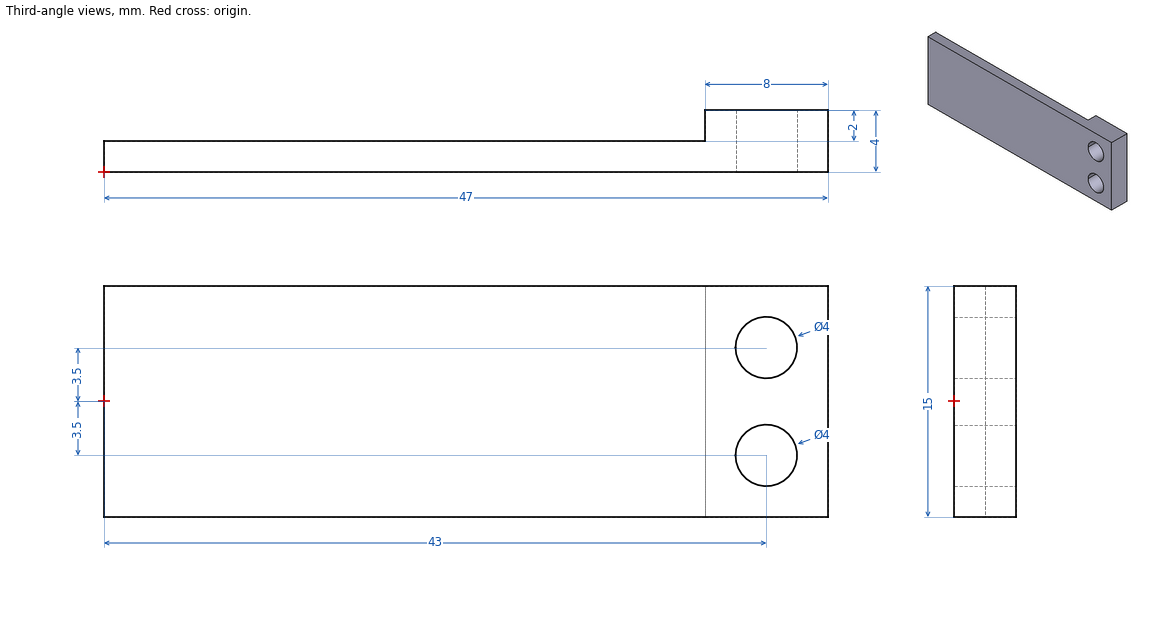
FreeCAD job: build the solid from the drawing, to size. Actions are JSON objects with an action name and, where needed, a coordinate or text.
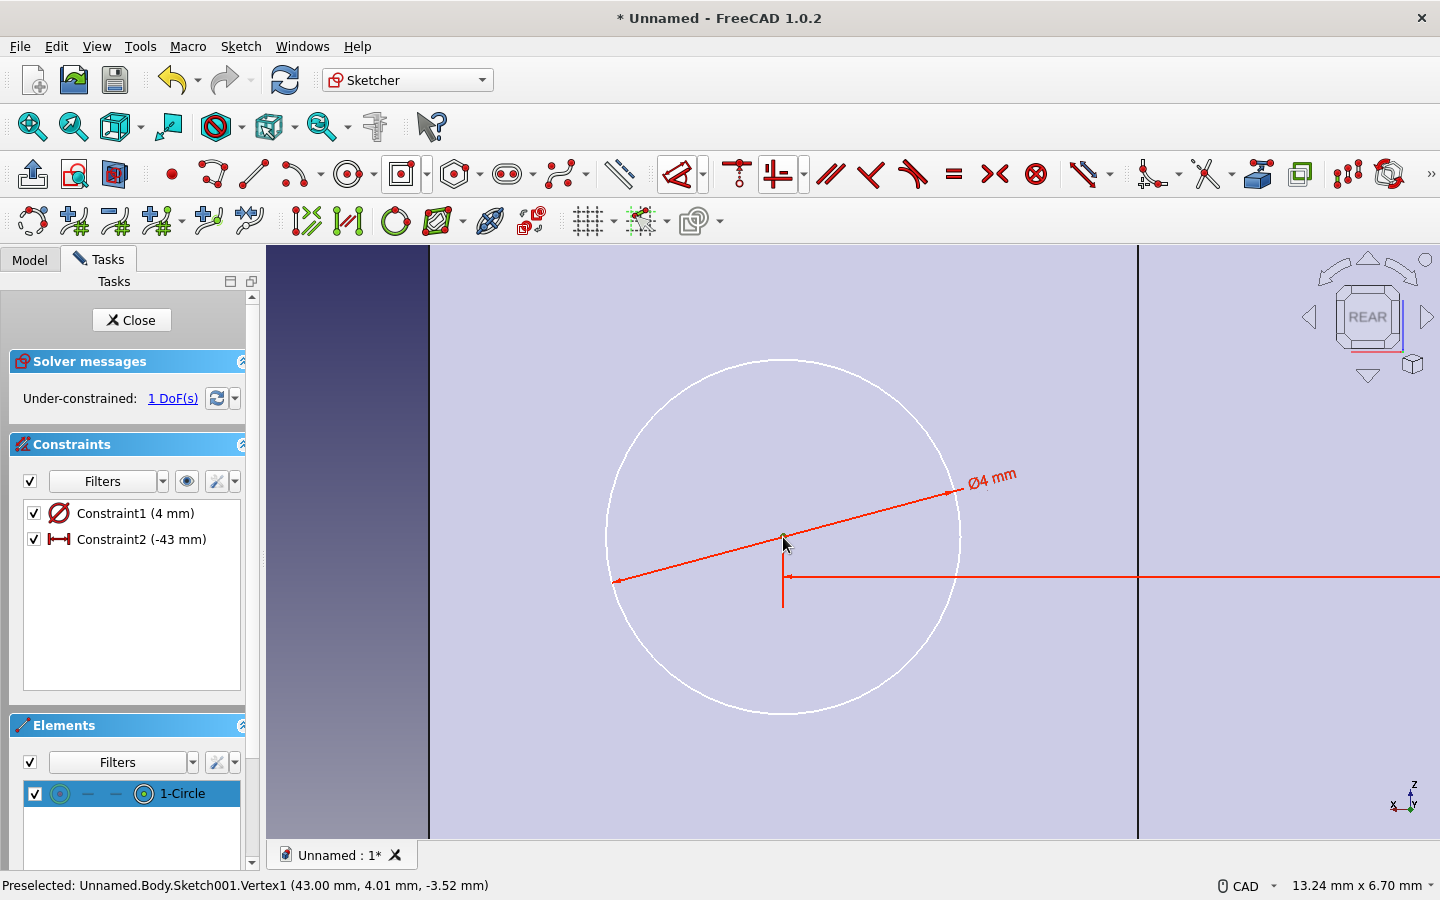
{"action": "left_click", "coordinate": [702, 174]}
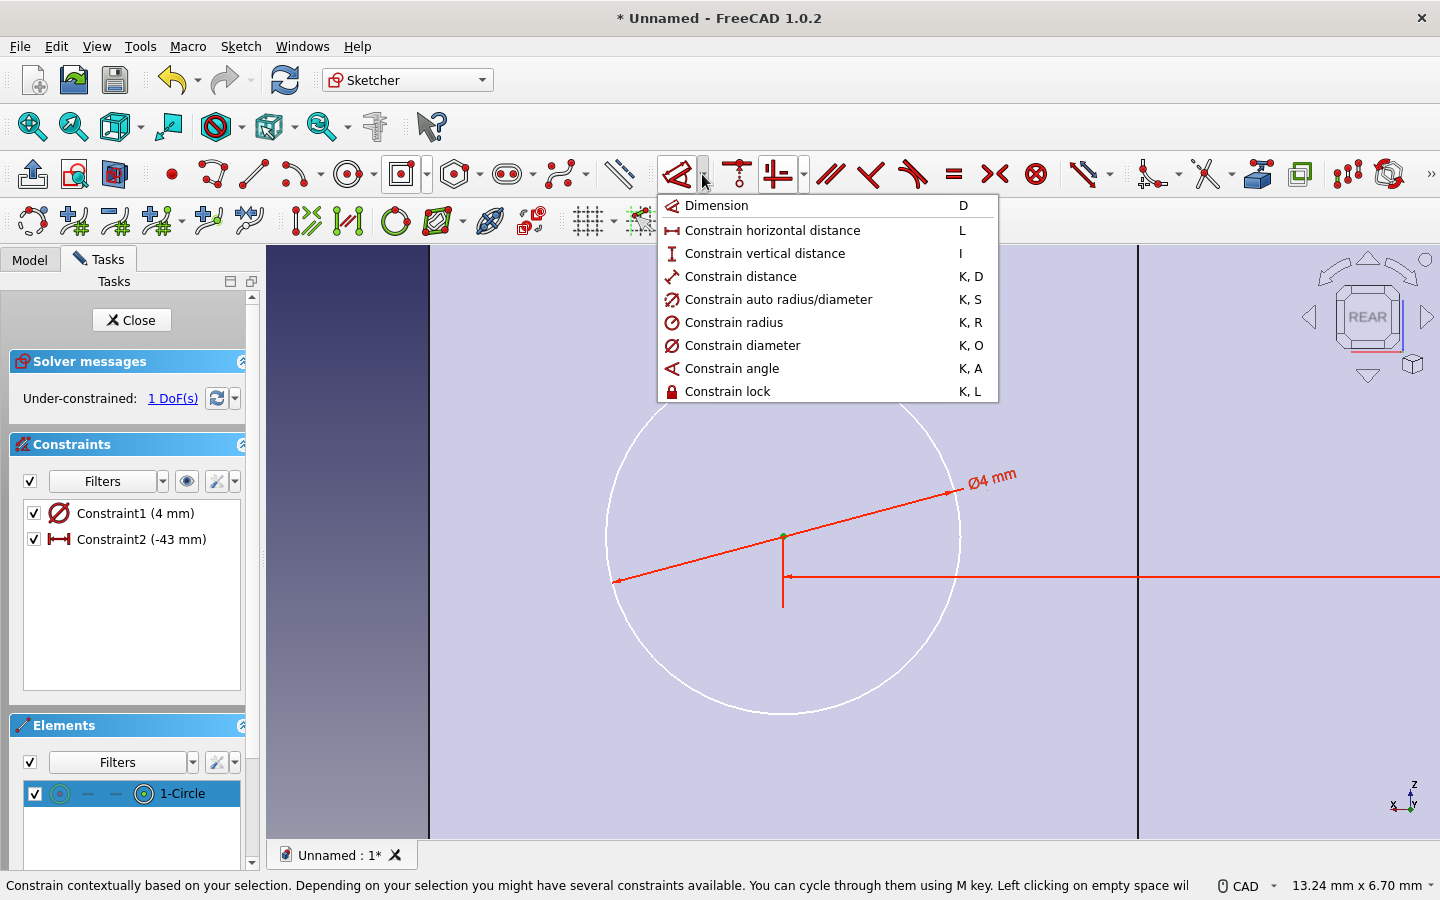
{"action": "left_click", "coordinate": [828, 254]}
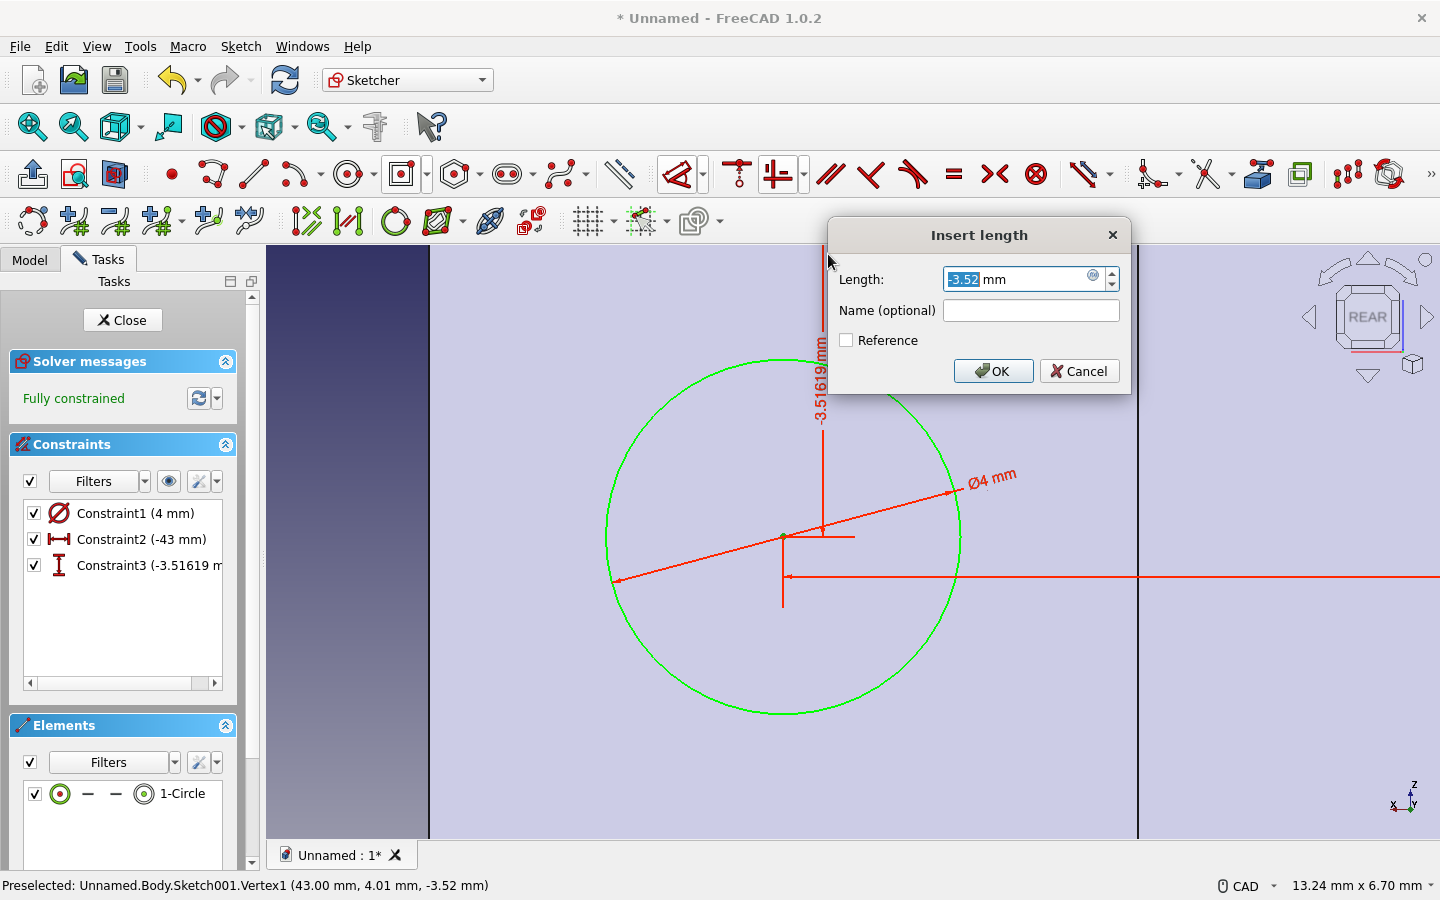
{"action": "type", "text": "-3.5"}
{"action": "key", "text": "Return"}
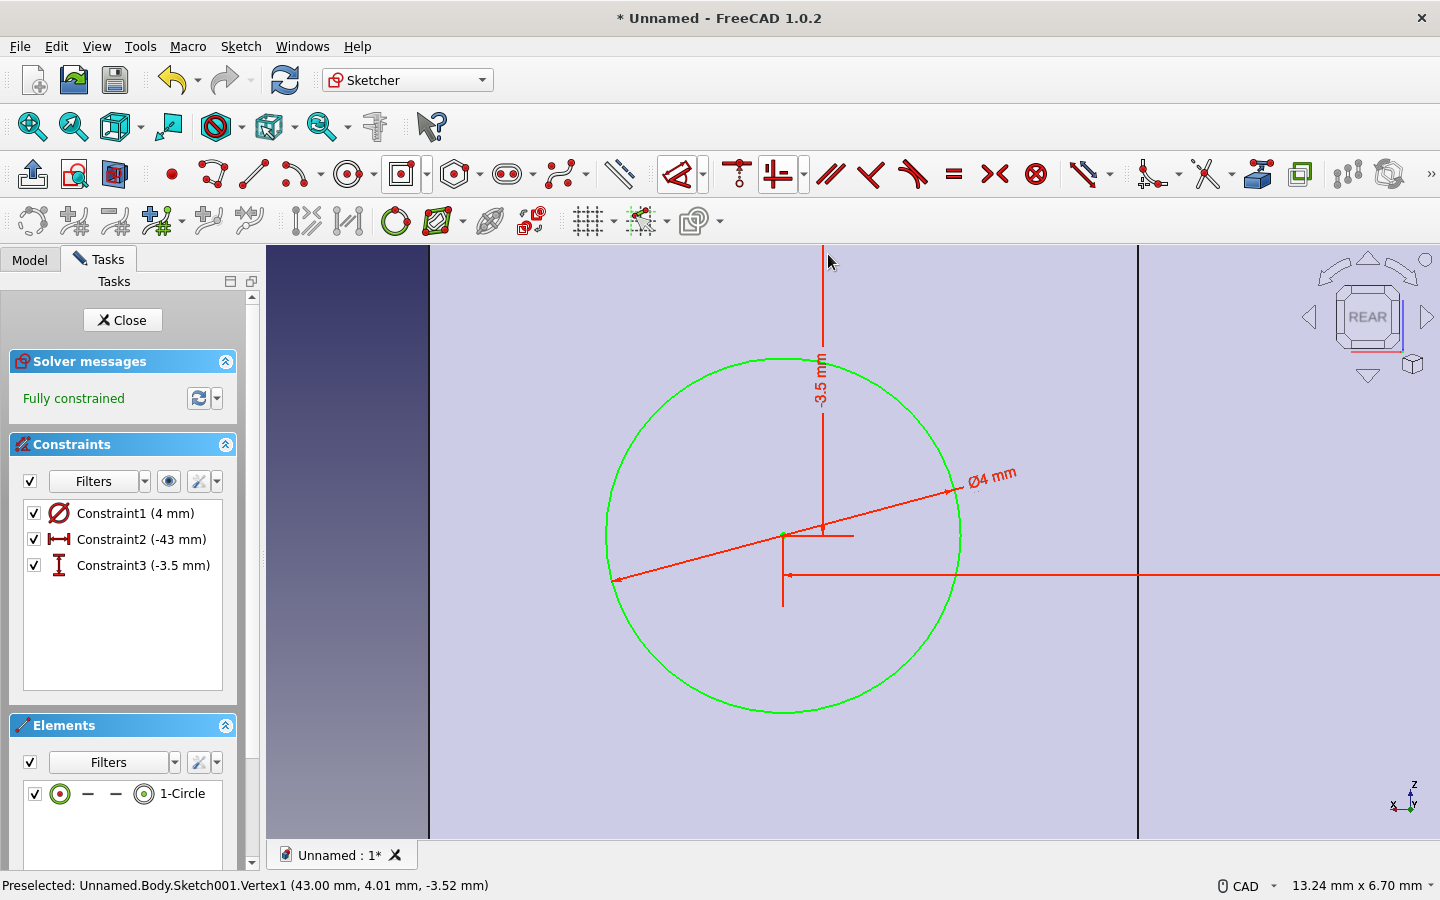
{"action": "left_click", "coordinate": [123, 320]}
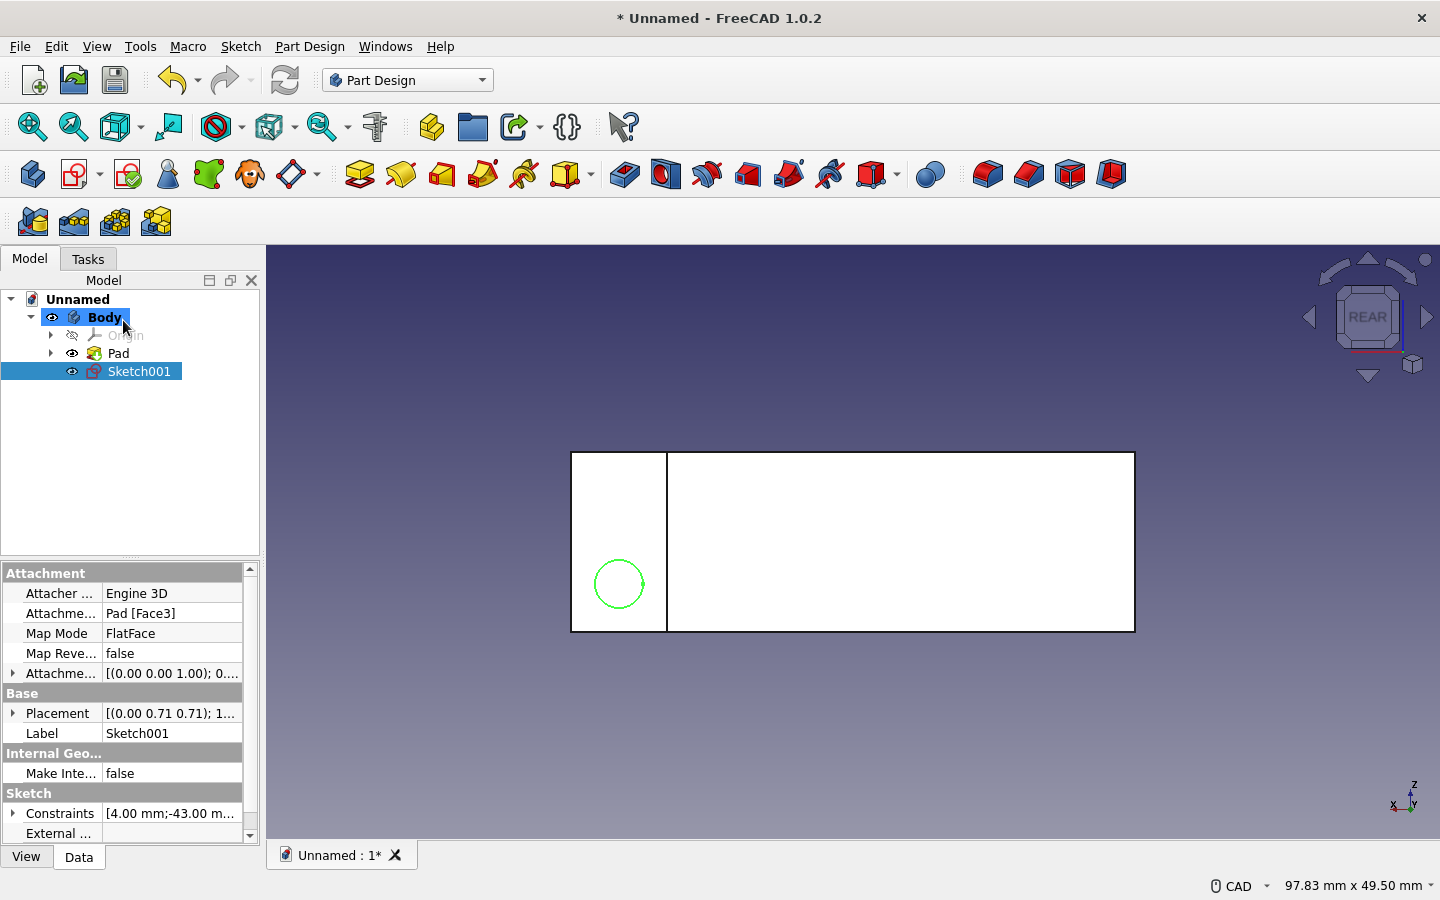
{"action": "left_click", "coordinate": [625, 174]}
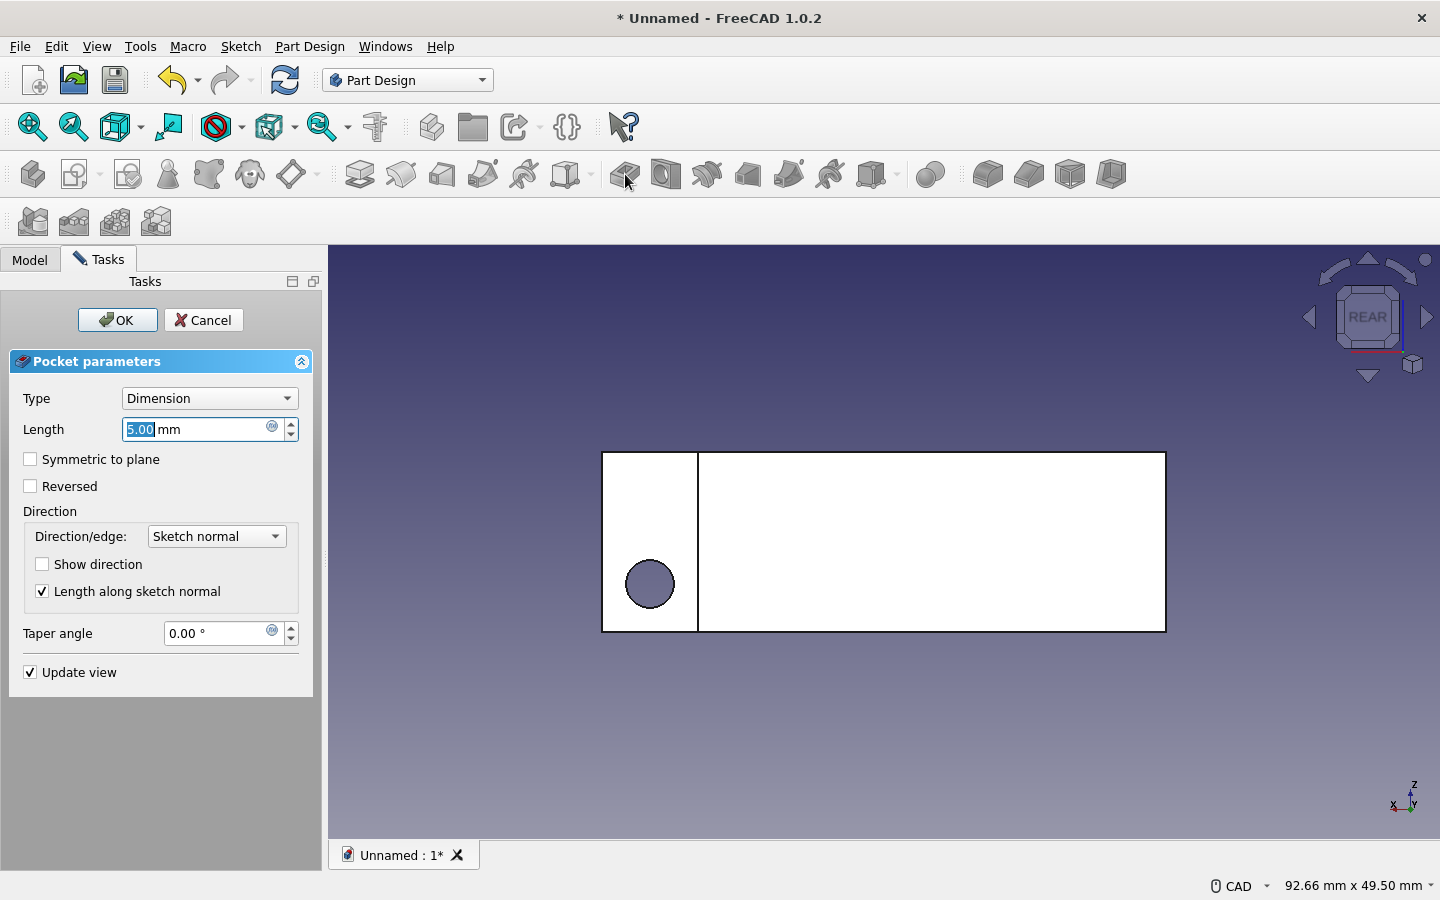
{"action": "left_click", "coordinate": [210, 398]}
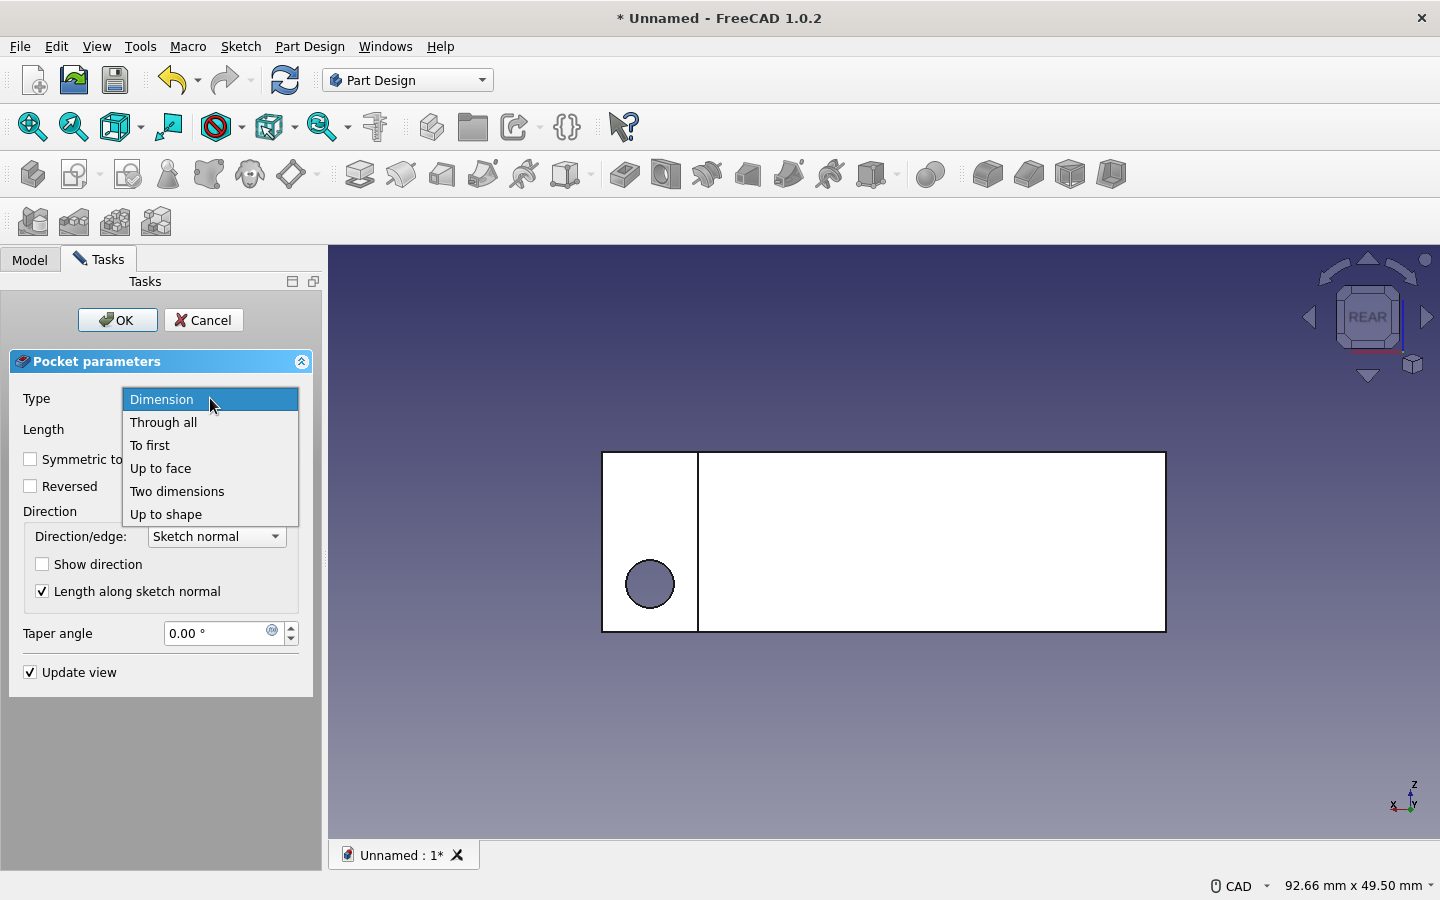
{"action": "left_click", "coordinate": [208, 446]}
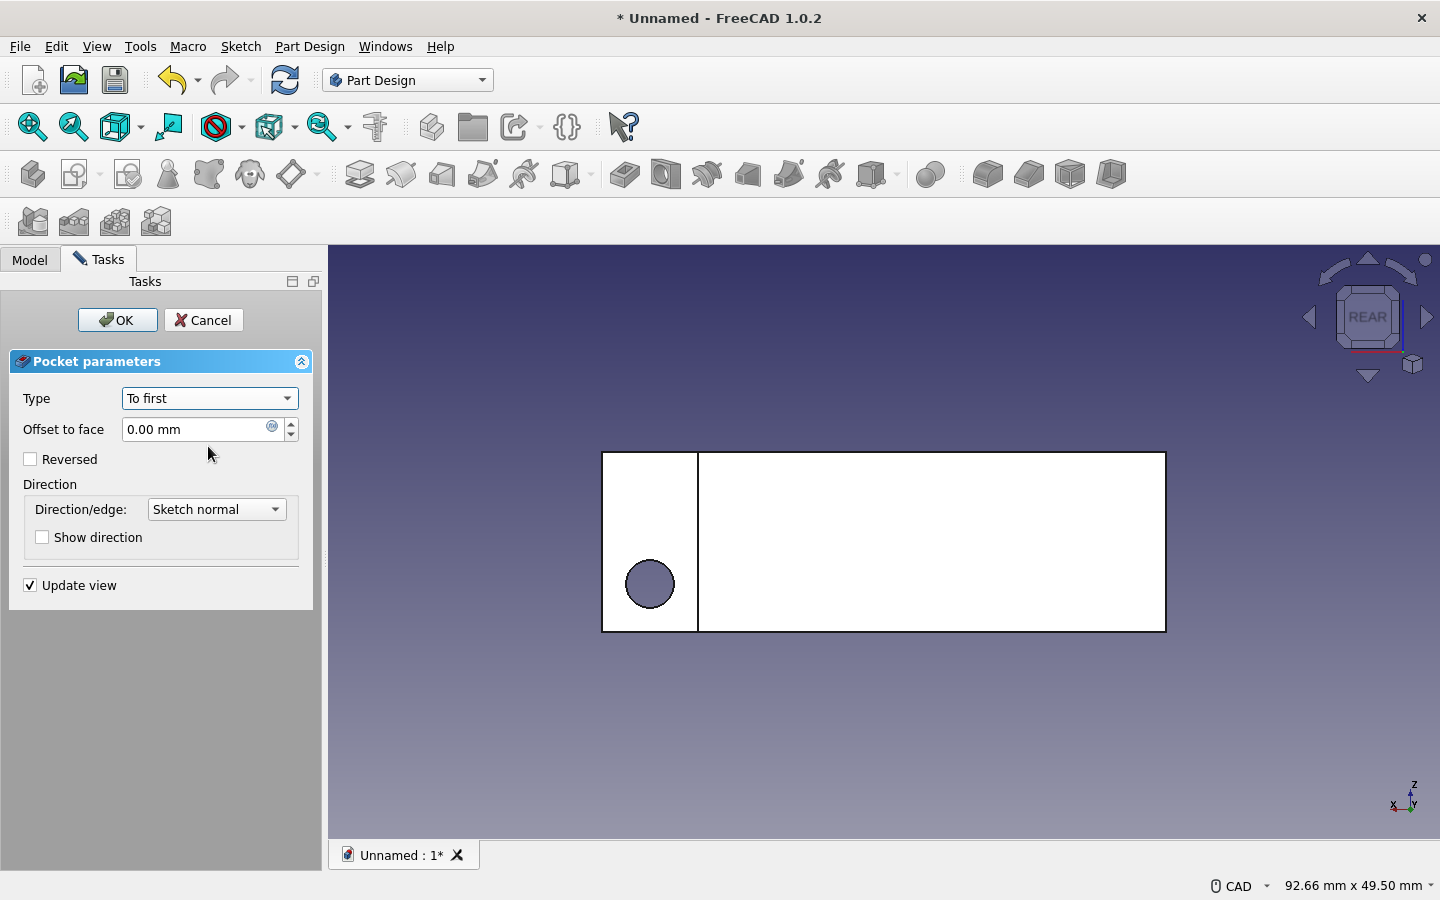
{"action": "left_click", "coordinate": [118, 320]}